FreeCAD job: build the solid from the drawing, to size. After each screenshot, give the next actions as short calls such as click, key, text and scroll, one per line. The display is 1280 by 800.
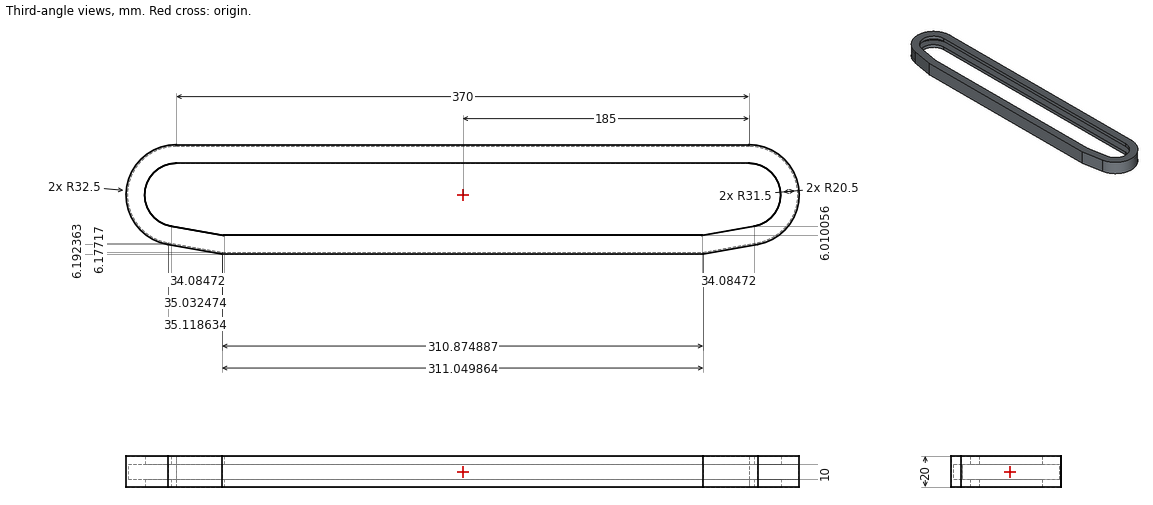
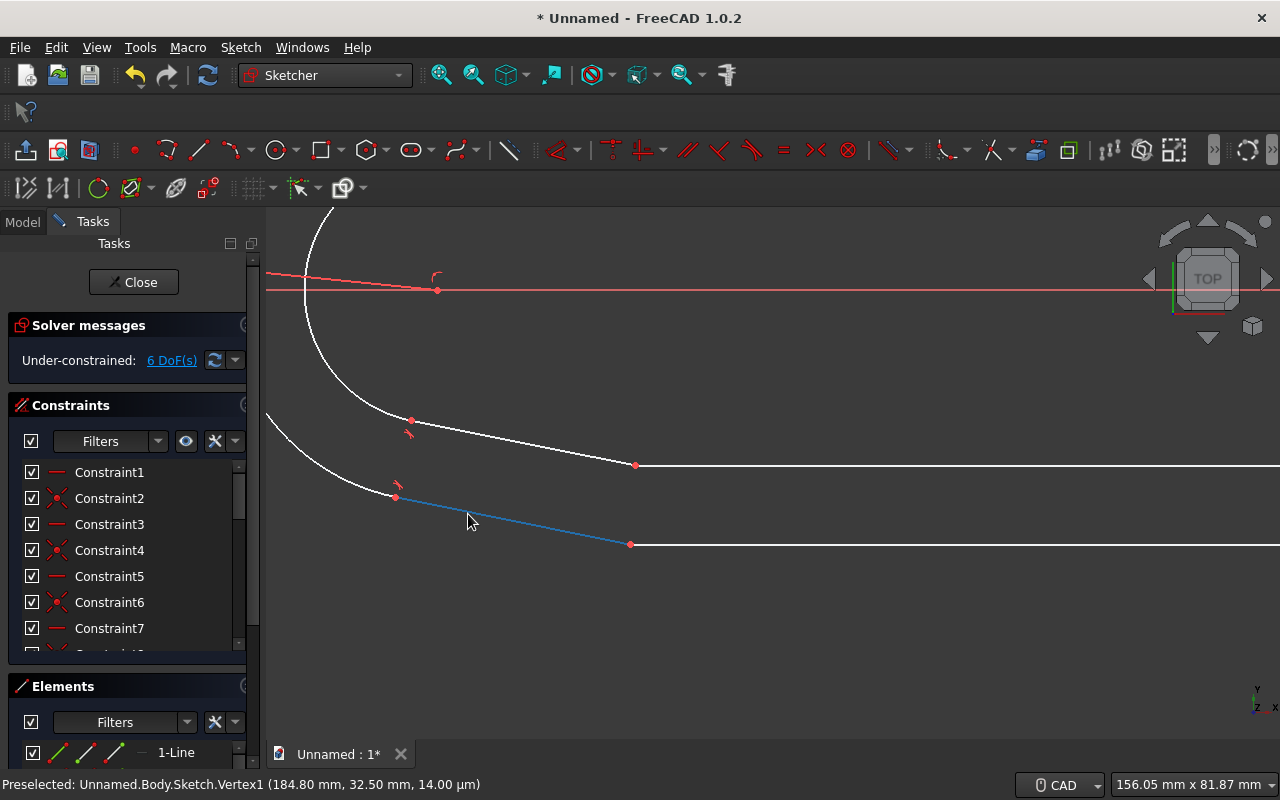
click(466, 511)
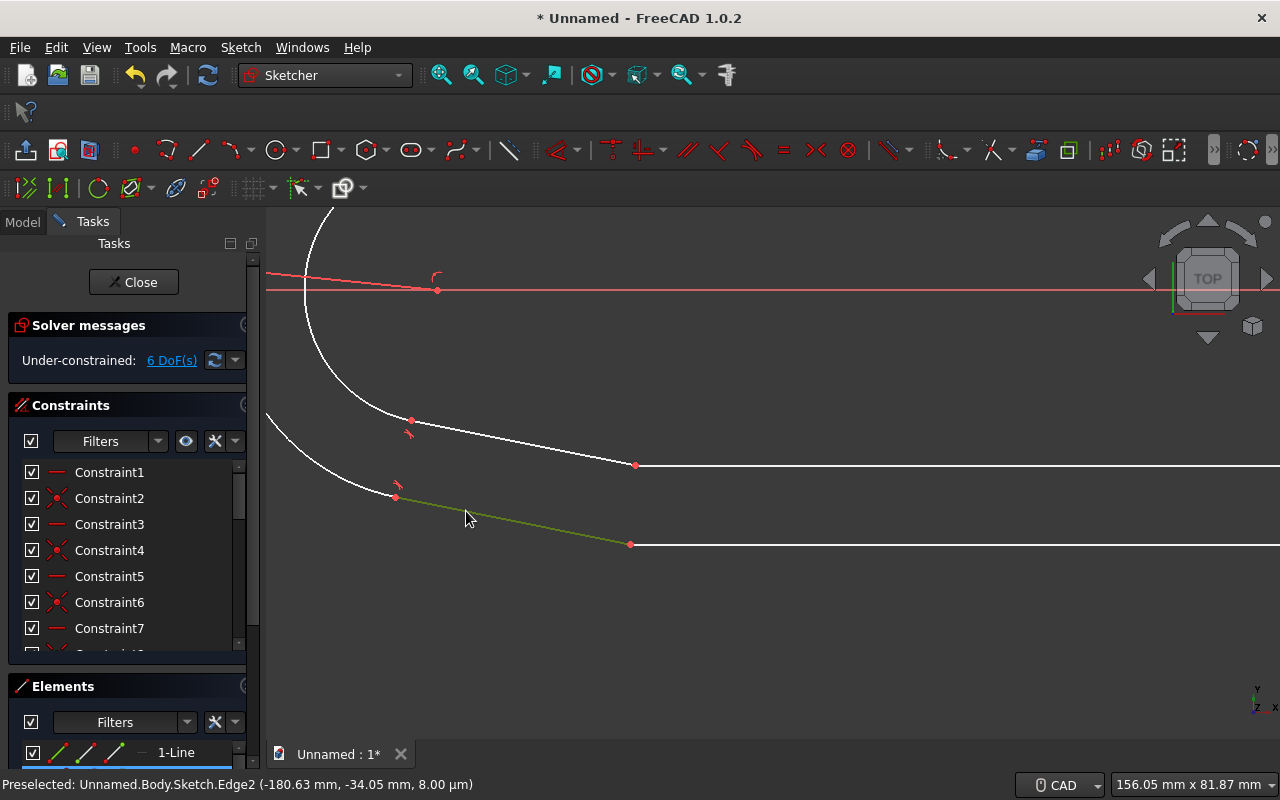
key(i)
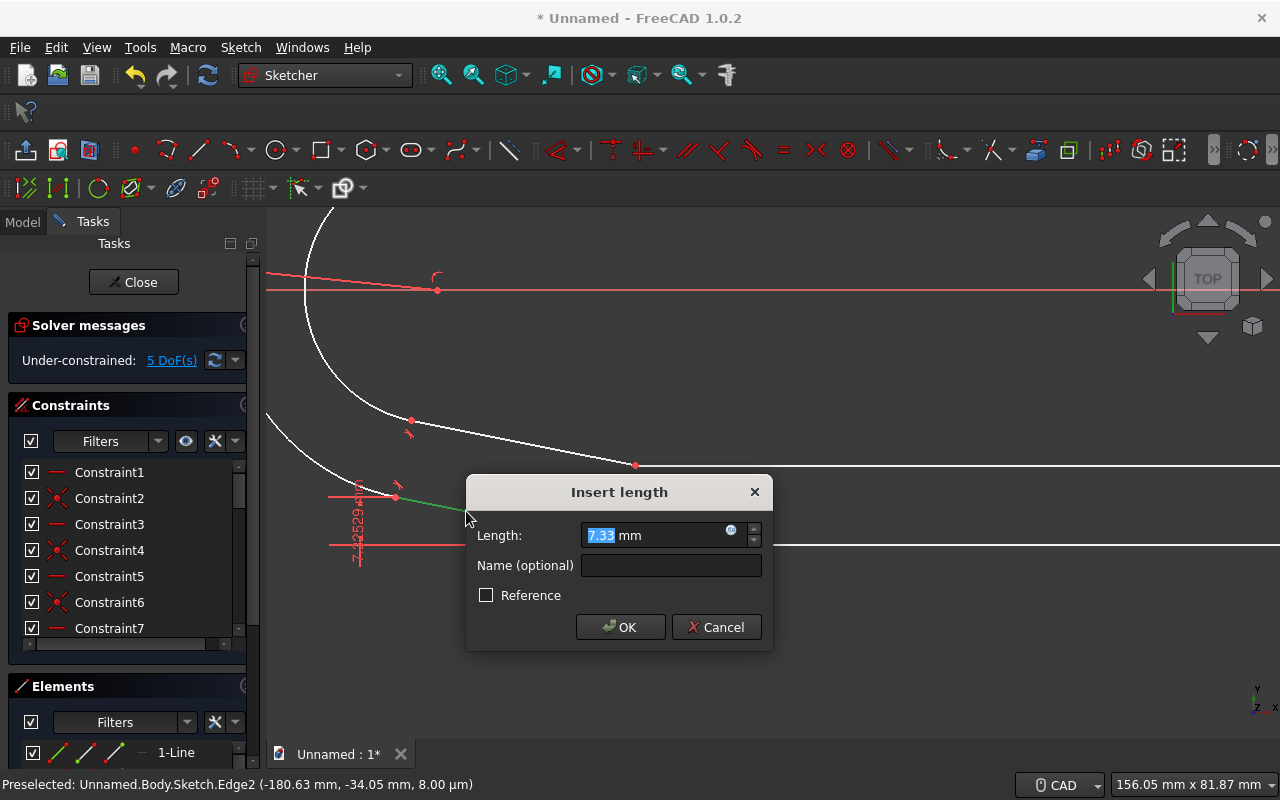
text(6.192363)
key(Return)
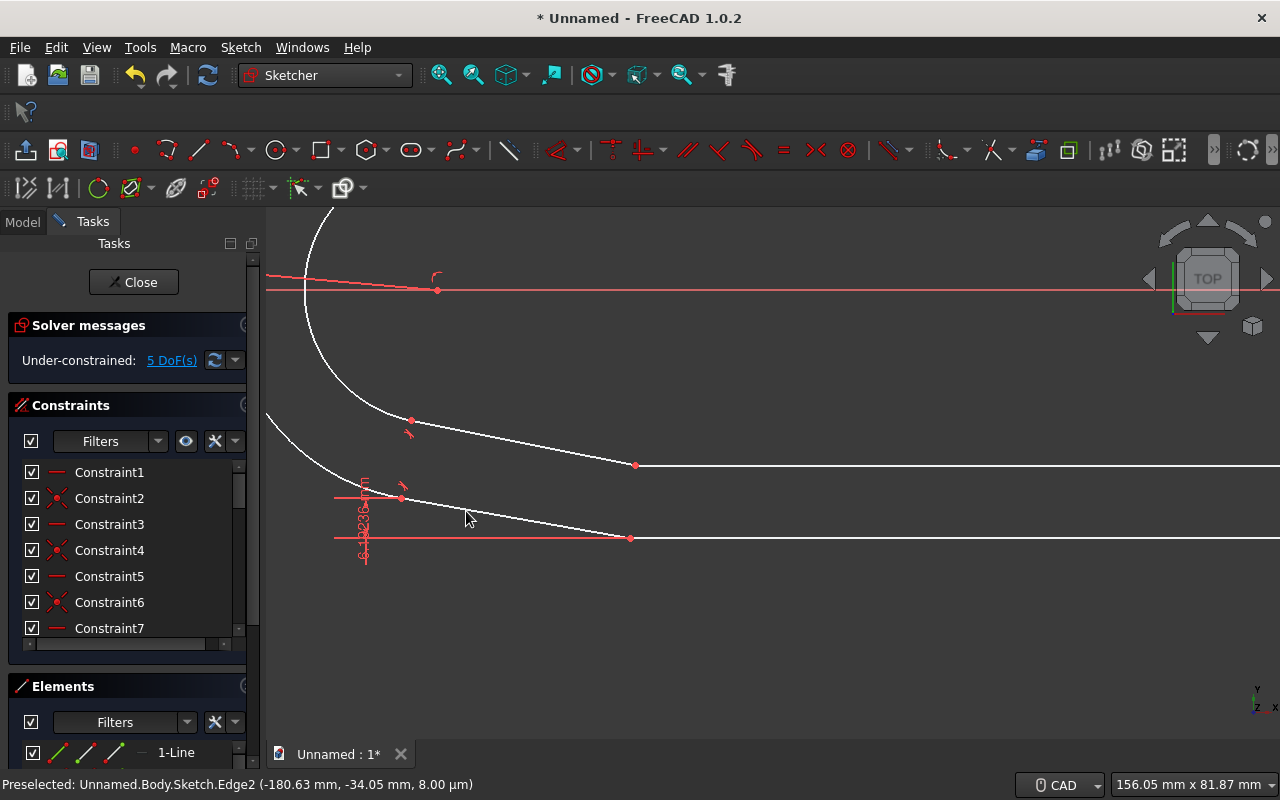
scroll(468, 515, down, 8)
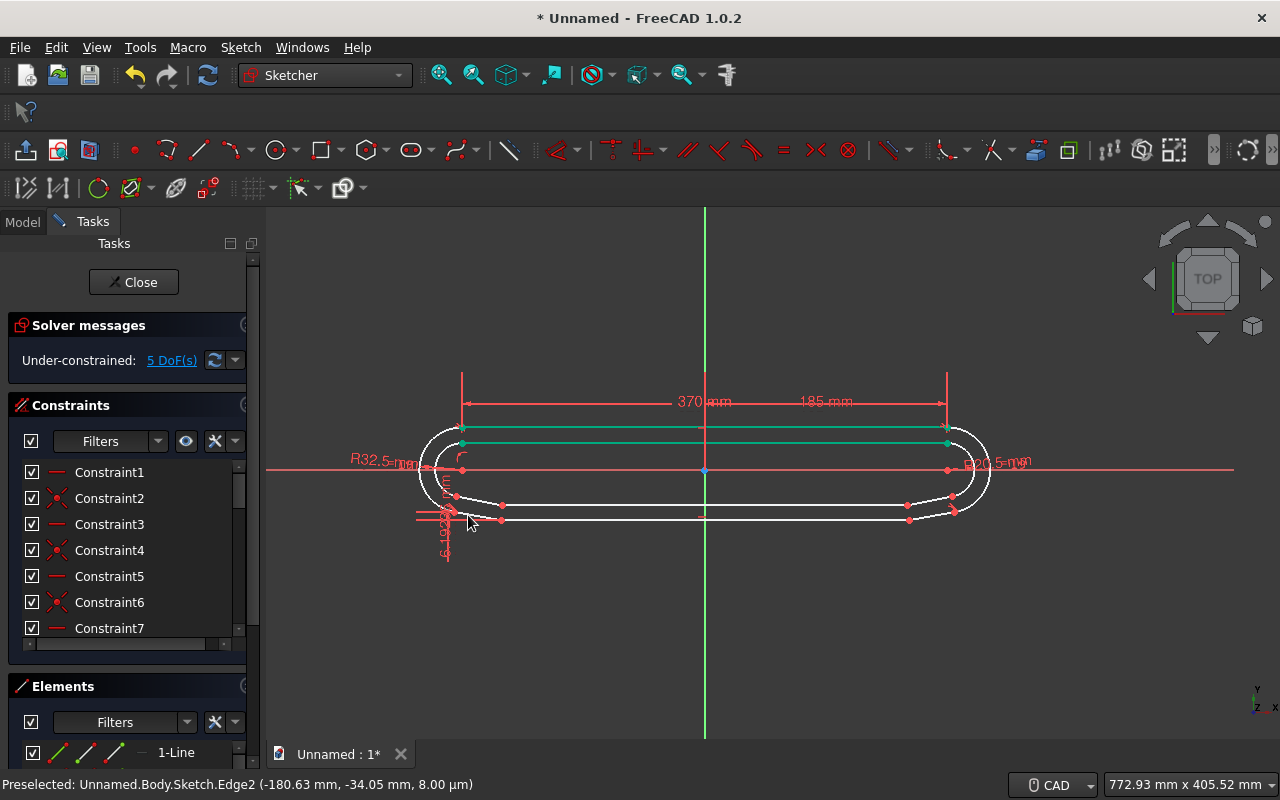
click(939, 499)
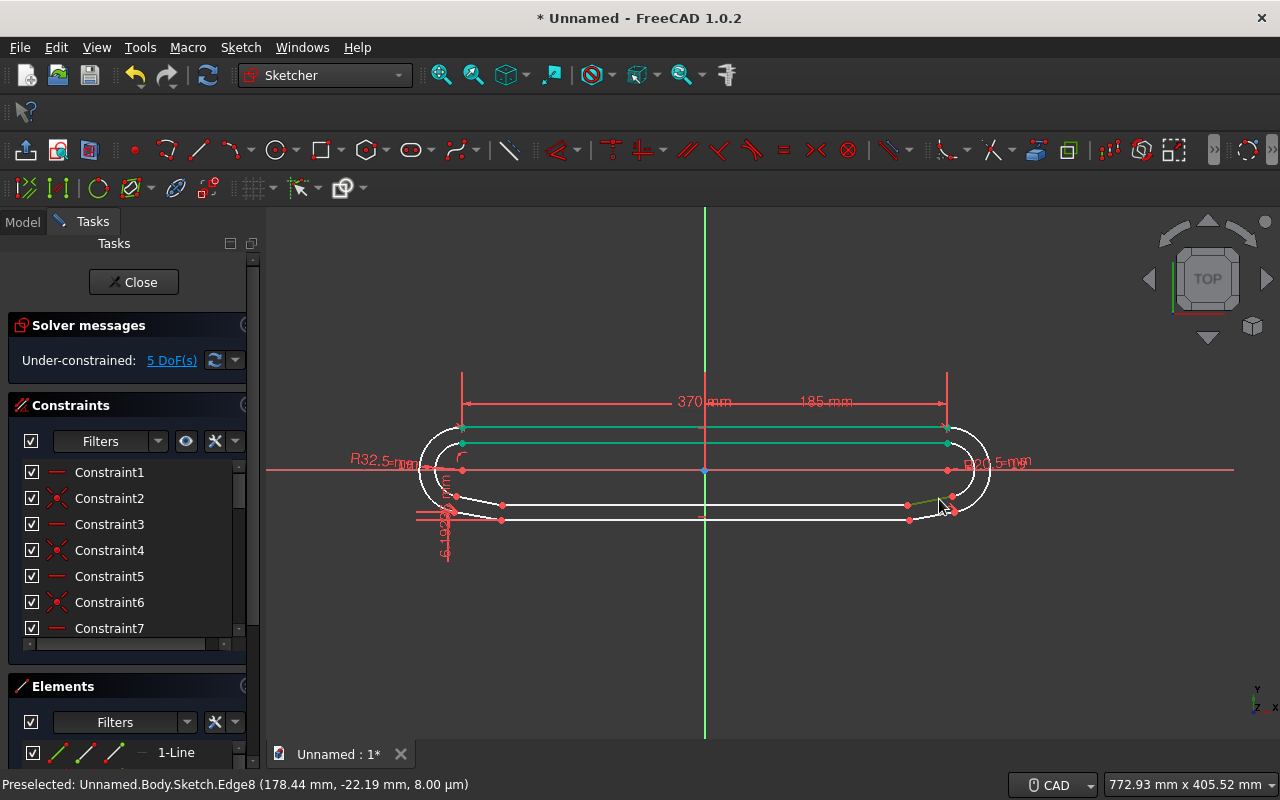
key(l)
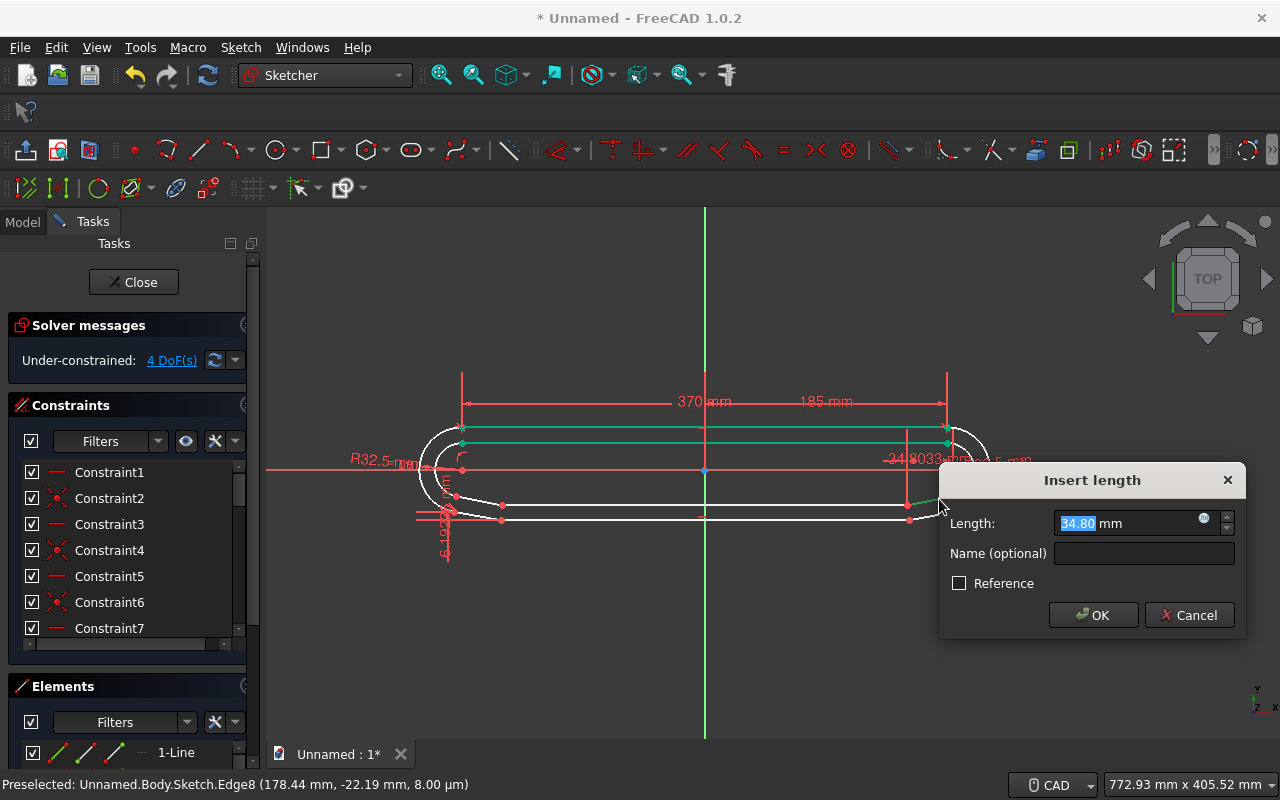
text(34.08472)
key(Return)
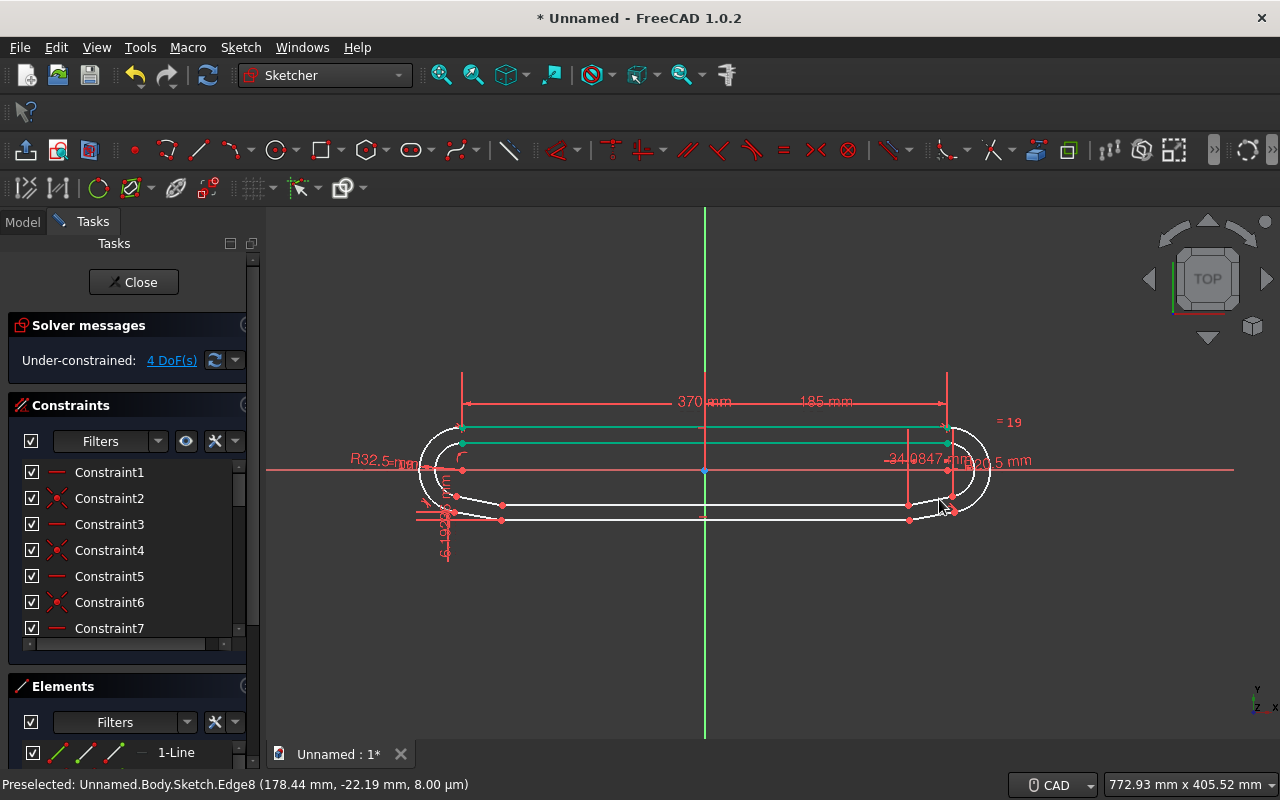
scroll(939, 499, up, 9)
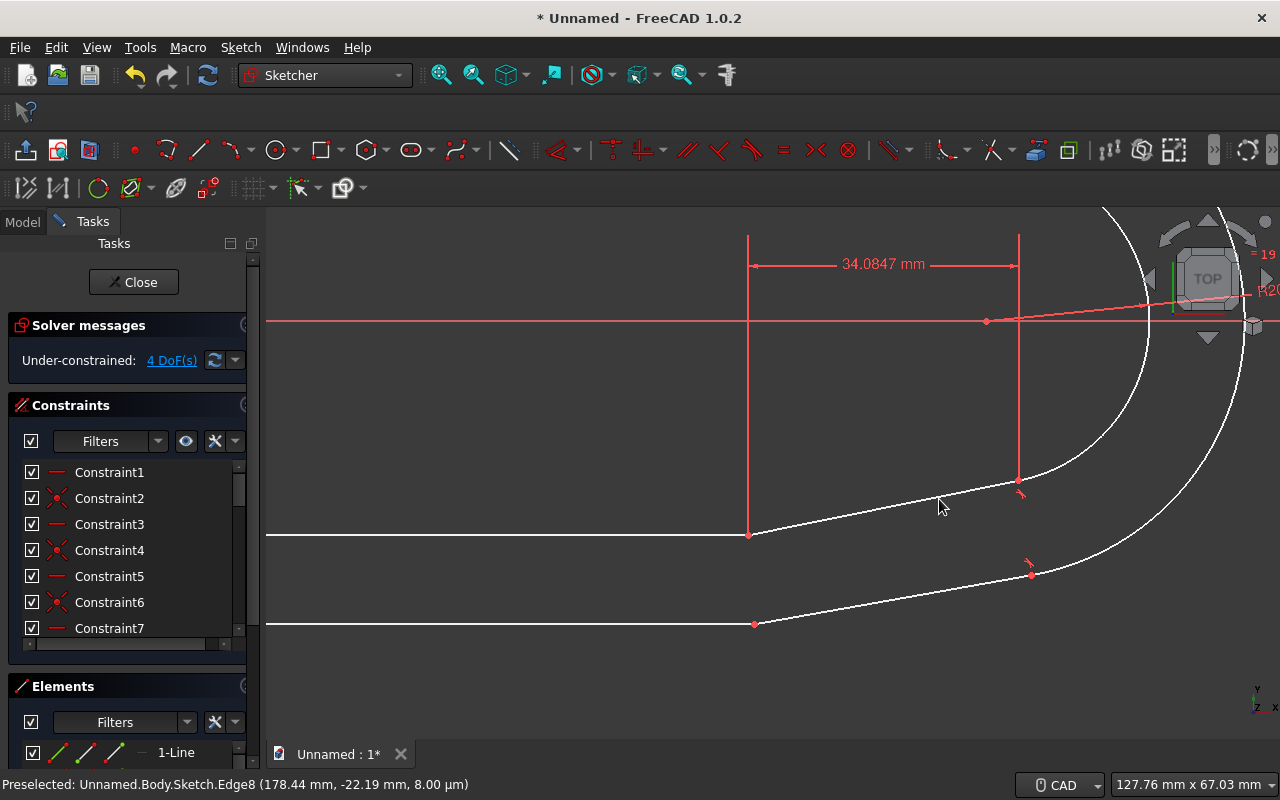
click(938, 497)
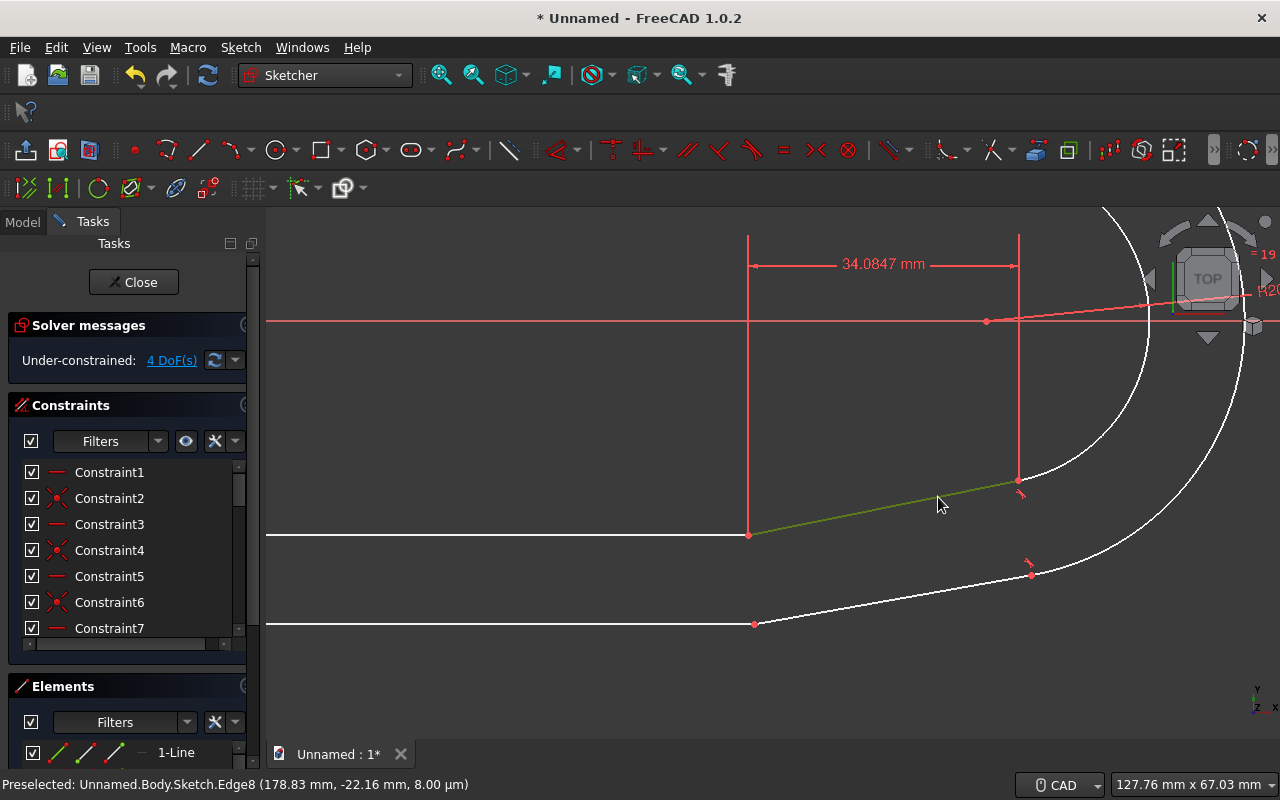
key(i)